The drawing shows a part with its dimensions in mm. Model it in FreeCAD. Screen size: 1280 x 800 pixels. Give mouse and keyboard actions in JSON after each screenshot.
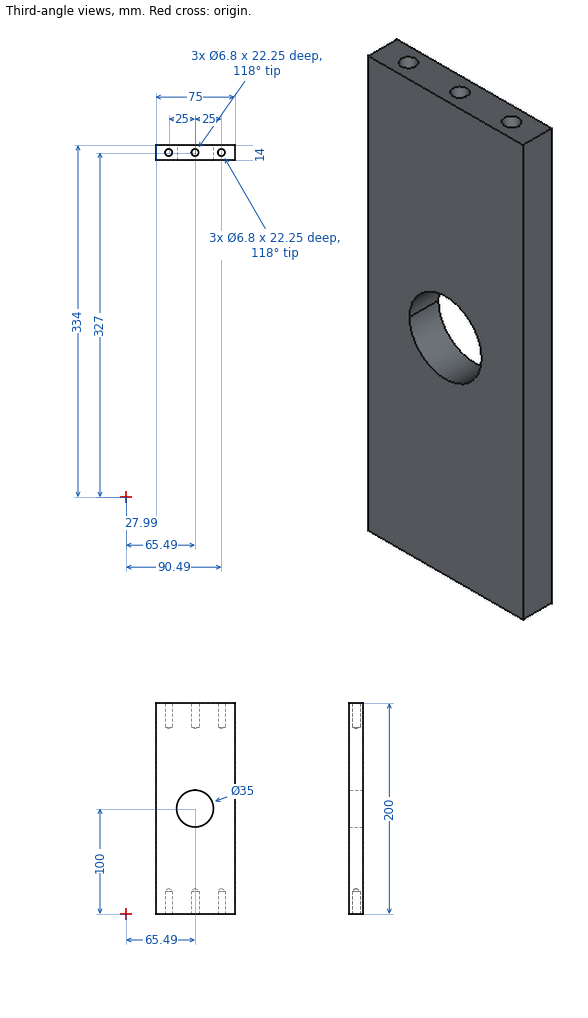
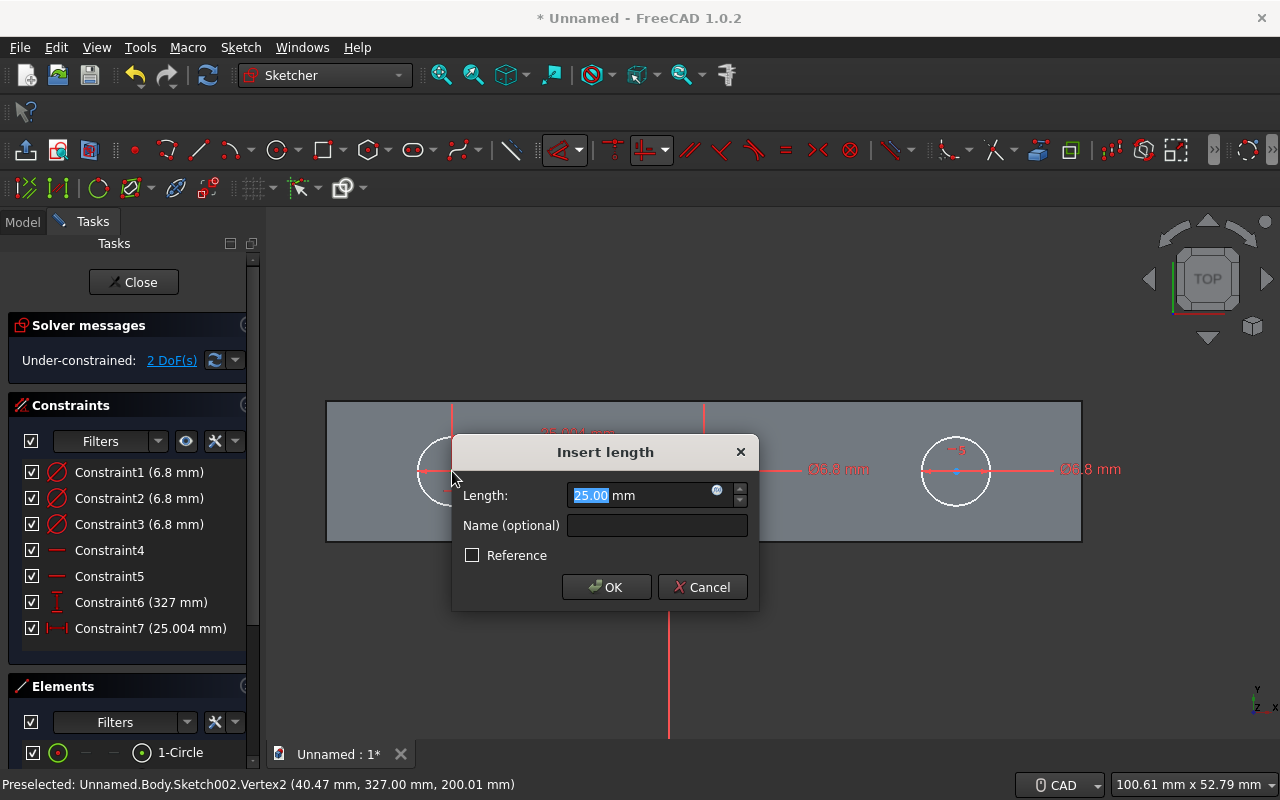
{"action": "type", "text": "25"}
{"action": "key", "text": "Return"}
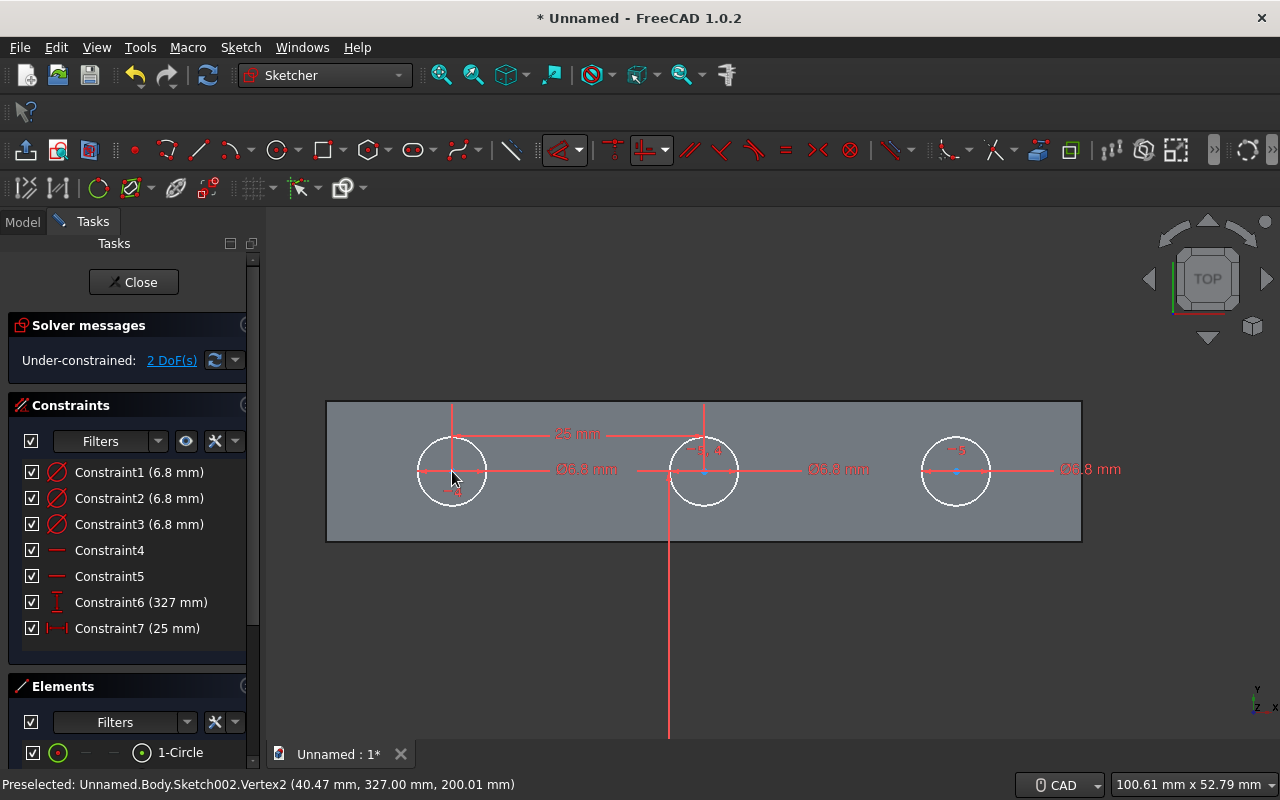
{"action": "left_click", "coordinate": [704, 471]}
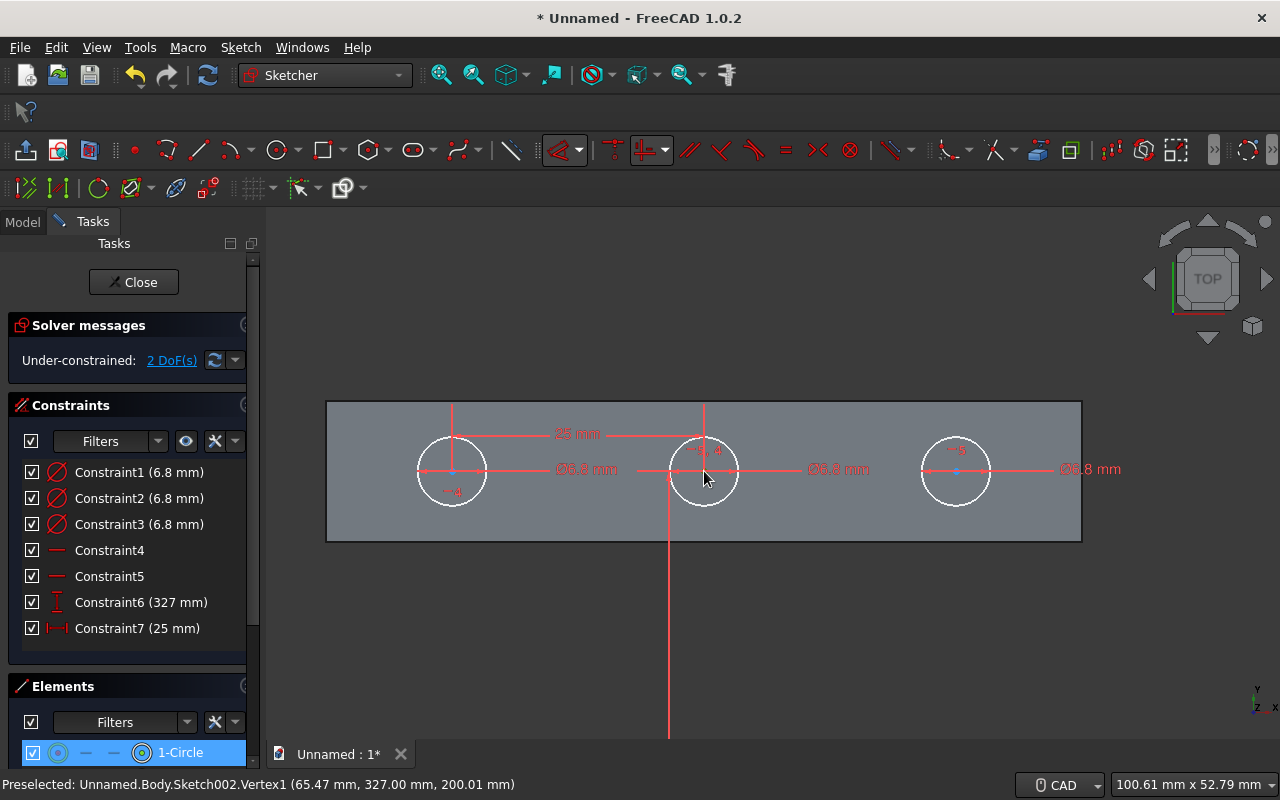
{"action": "left_click", "coordinate": [956, 471]}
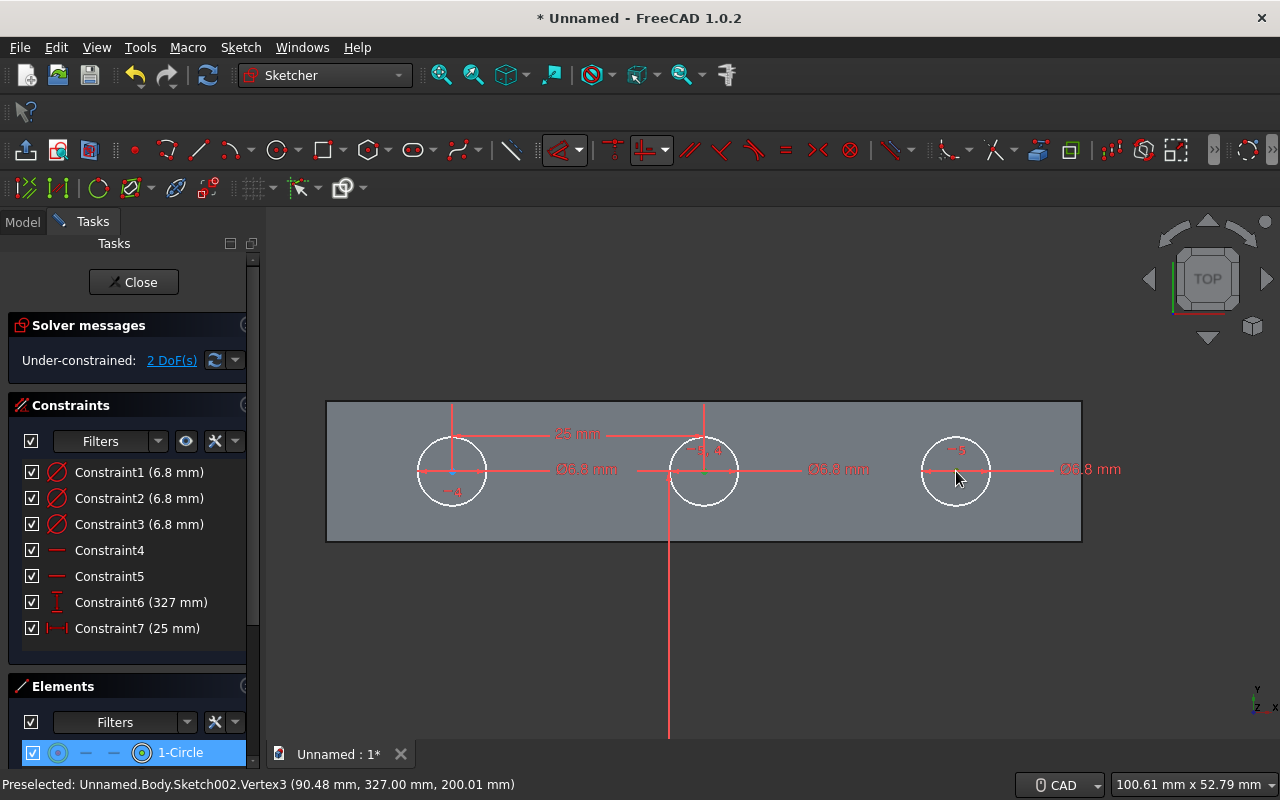
{"action": "key", "text": "l"}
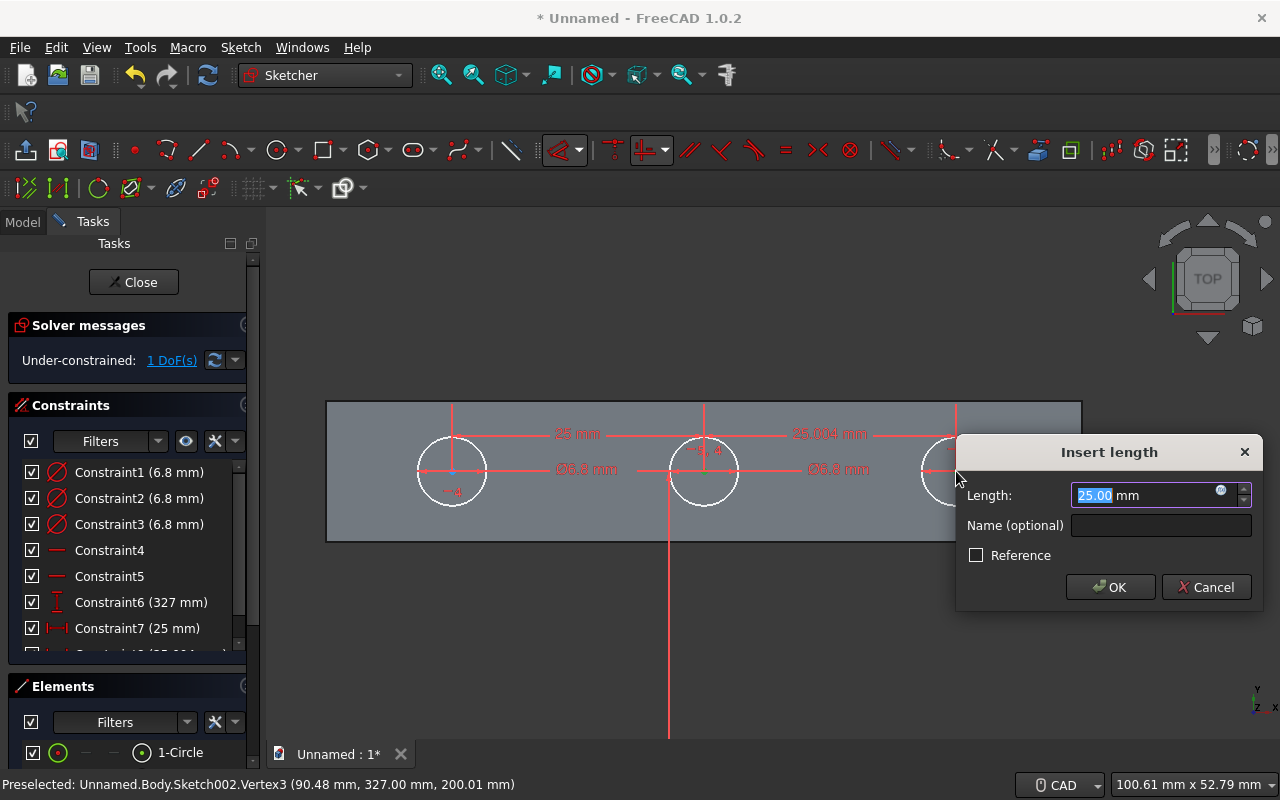
{"action": "type", "text": "25"}
{"action": "key", "text": "Return"}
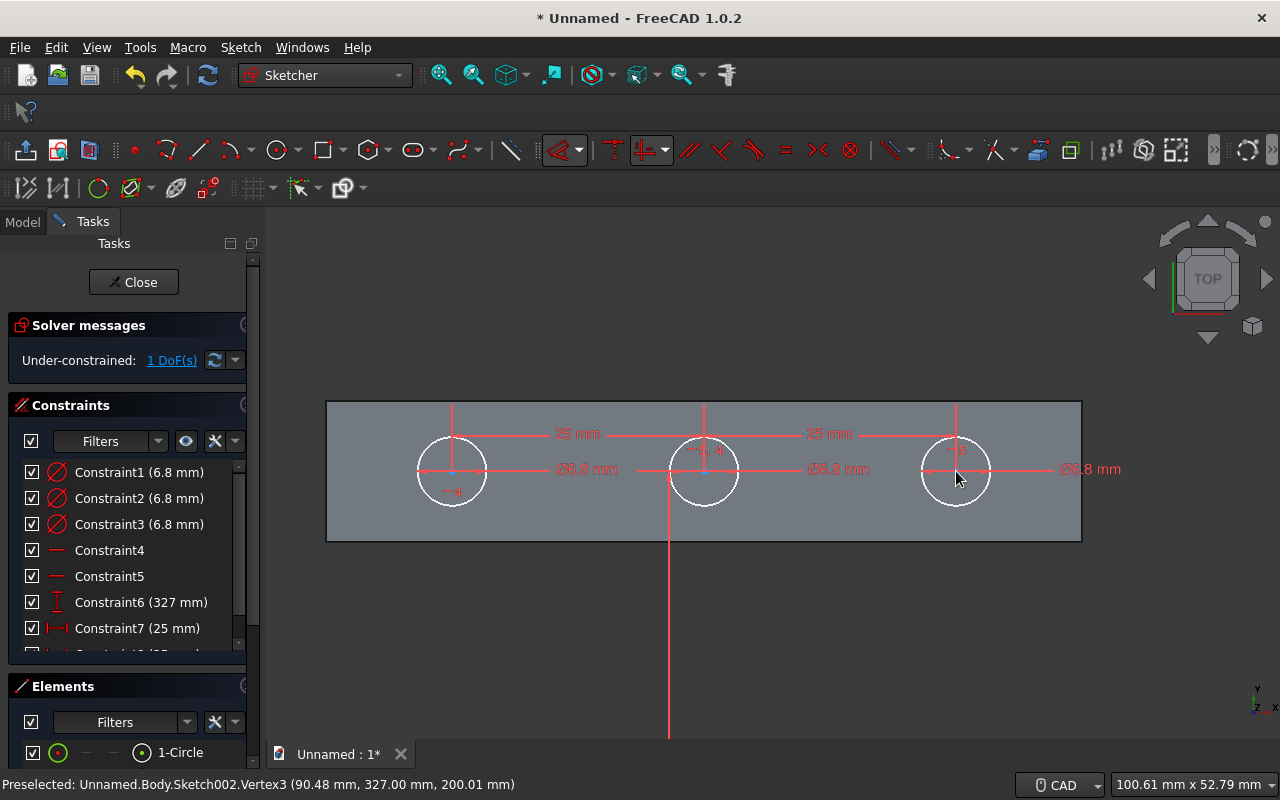
{"action": "left_click", "coordinate": [704, 471]}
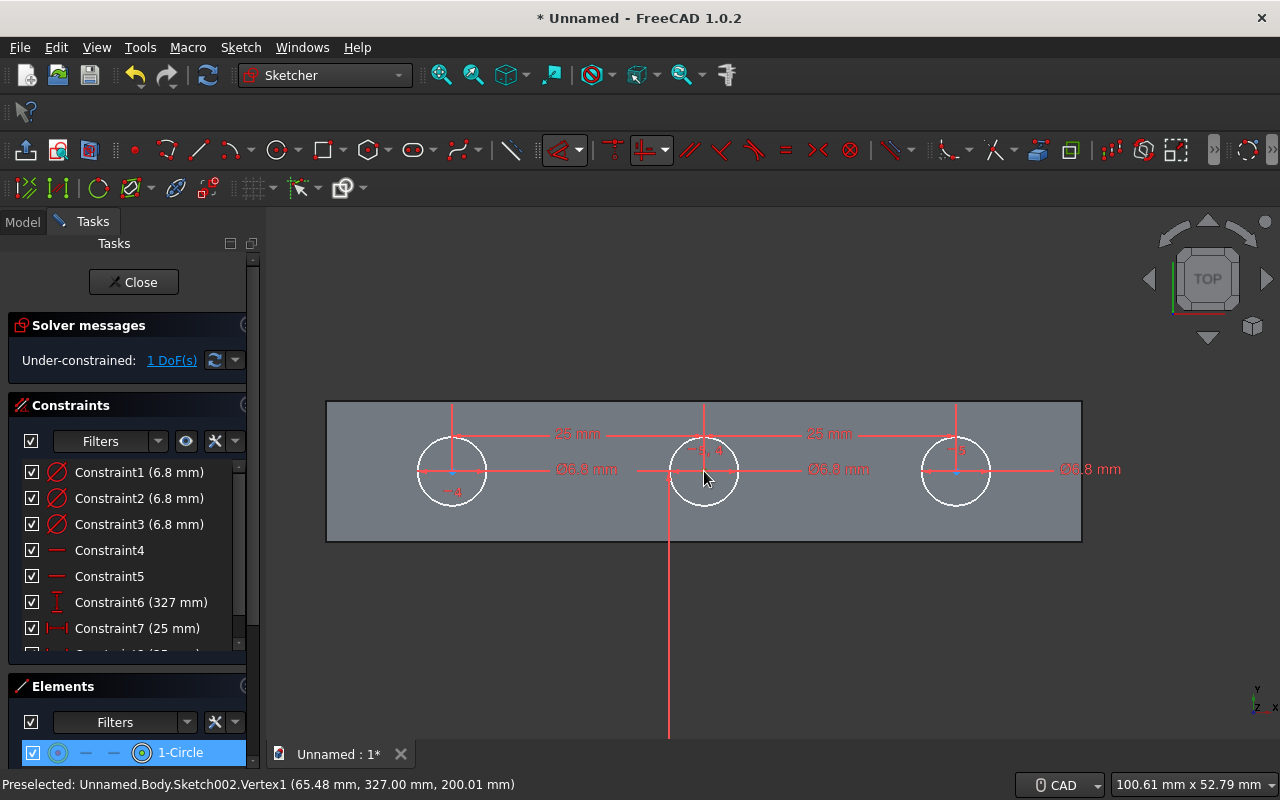
{"action": "left_click", "coordinate": [582, 150]}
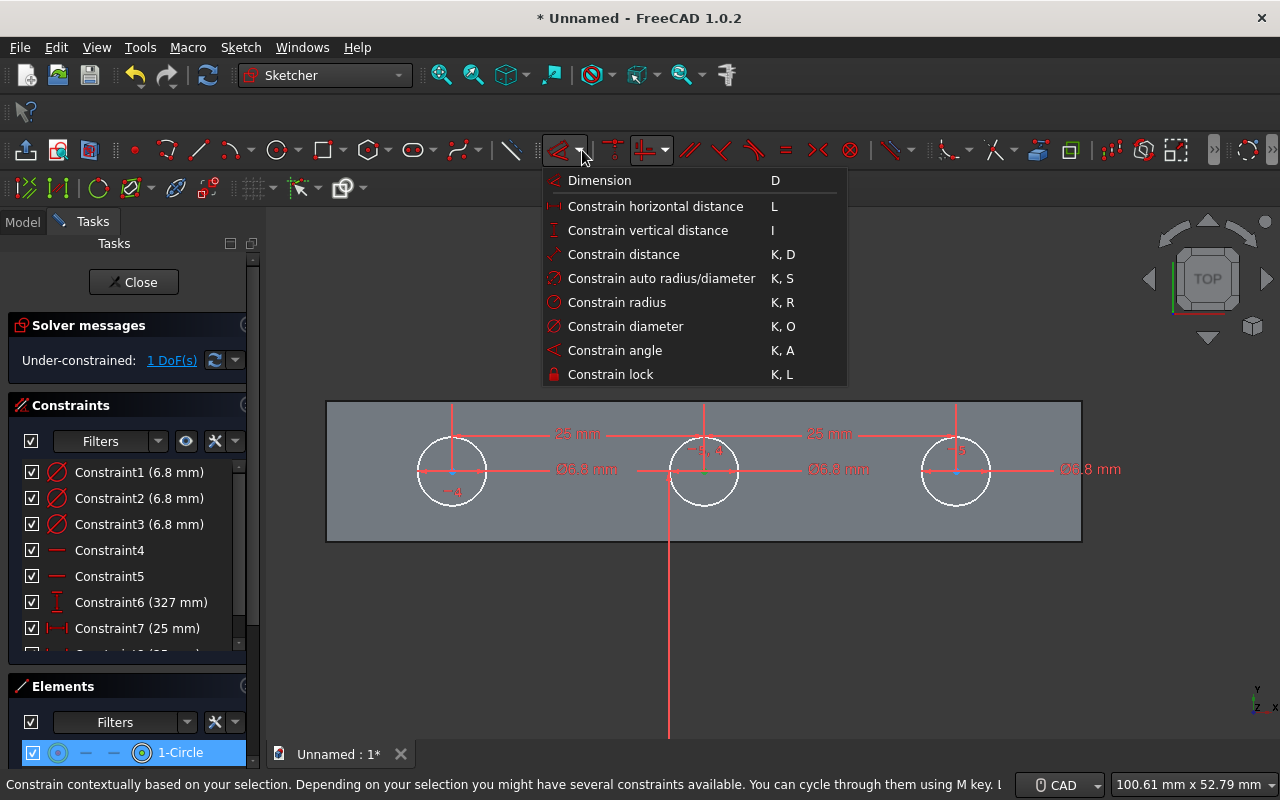
{"action": "left_click", "coordinate": [695, 206]}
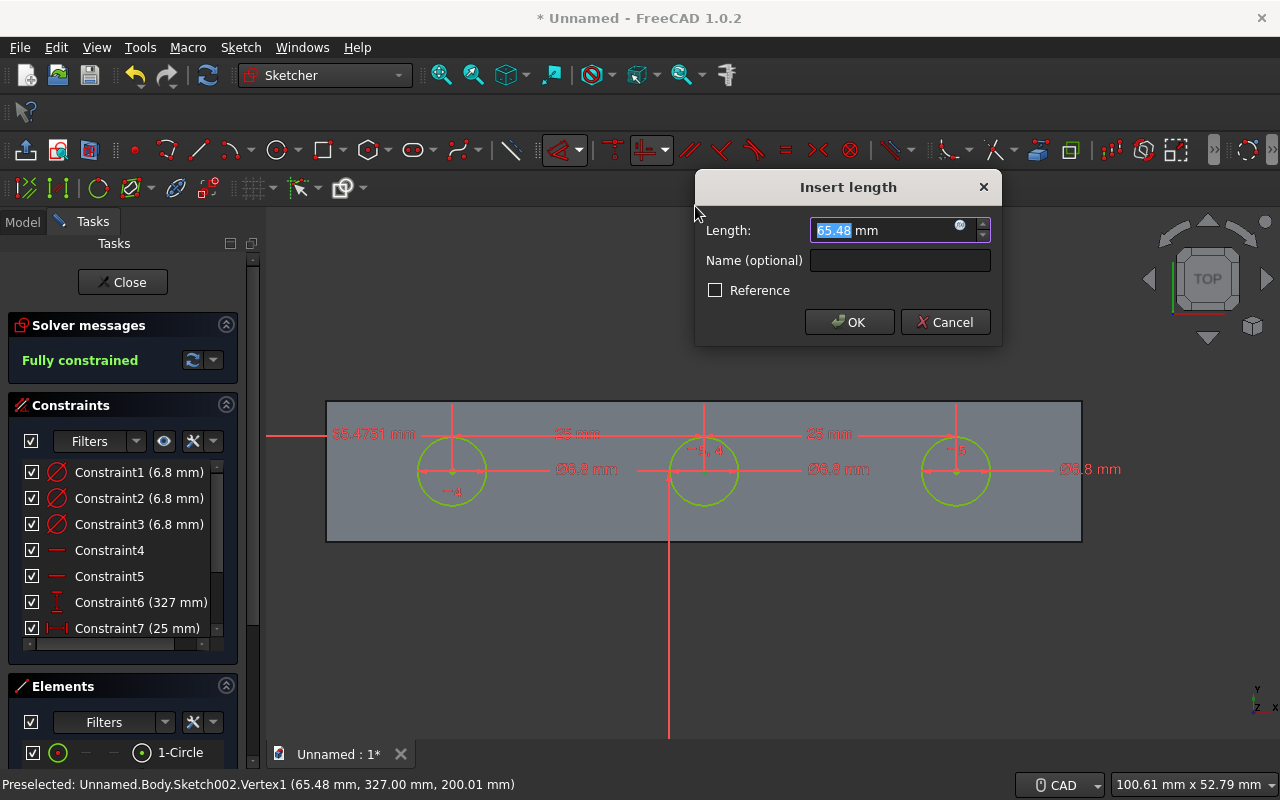
{"action": "type", "text": "65.49"}
{"action": "key", "text": "Return"}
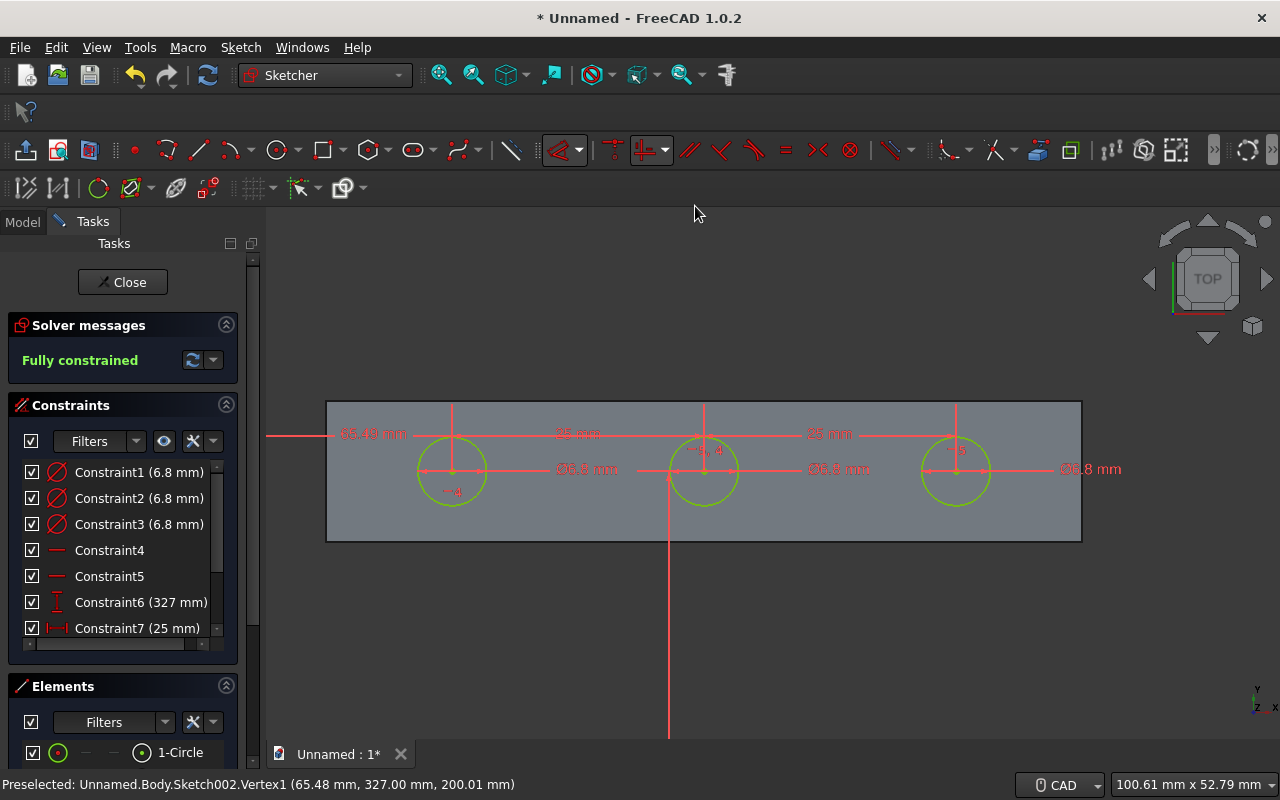
{"action": "left_click", "coordinate": [123, 282]}